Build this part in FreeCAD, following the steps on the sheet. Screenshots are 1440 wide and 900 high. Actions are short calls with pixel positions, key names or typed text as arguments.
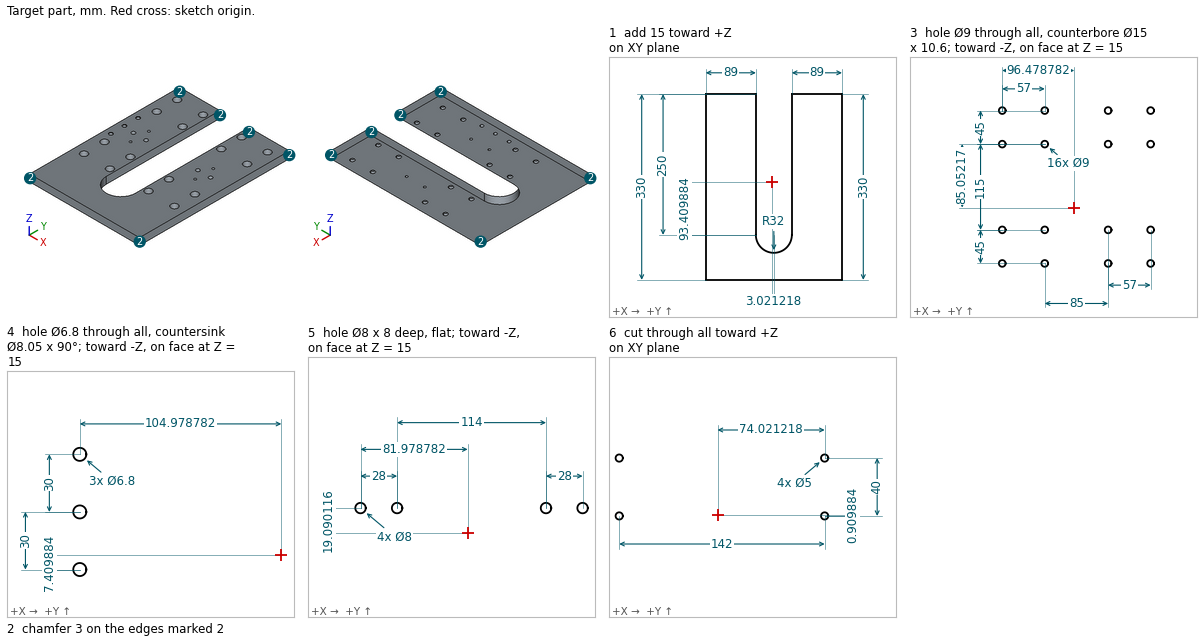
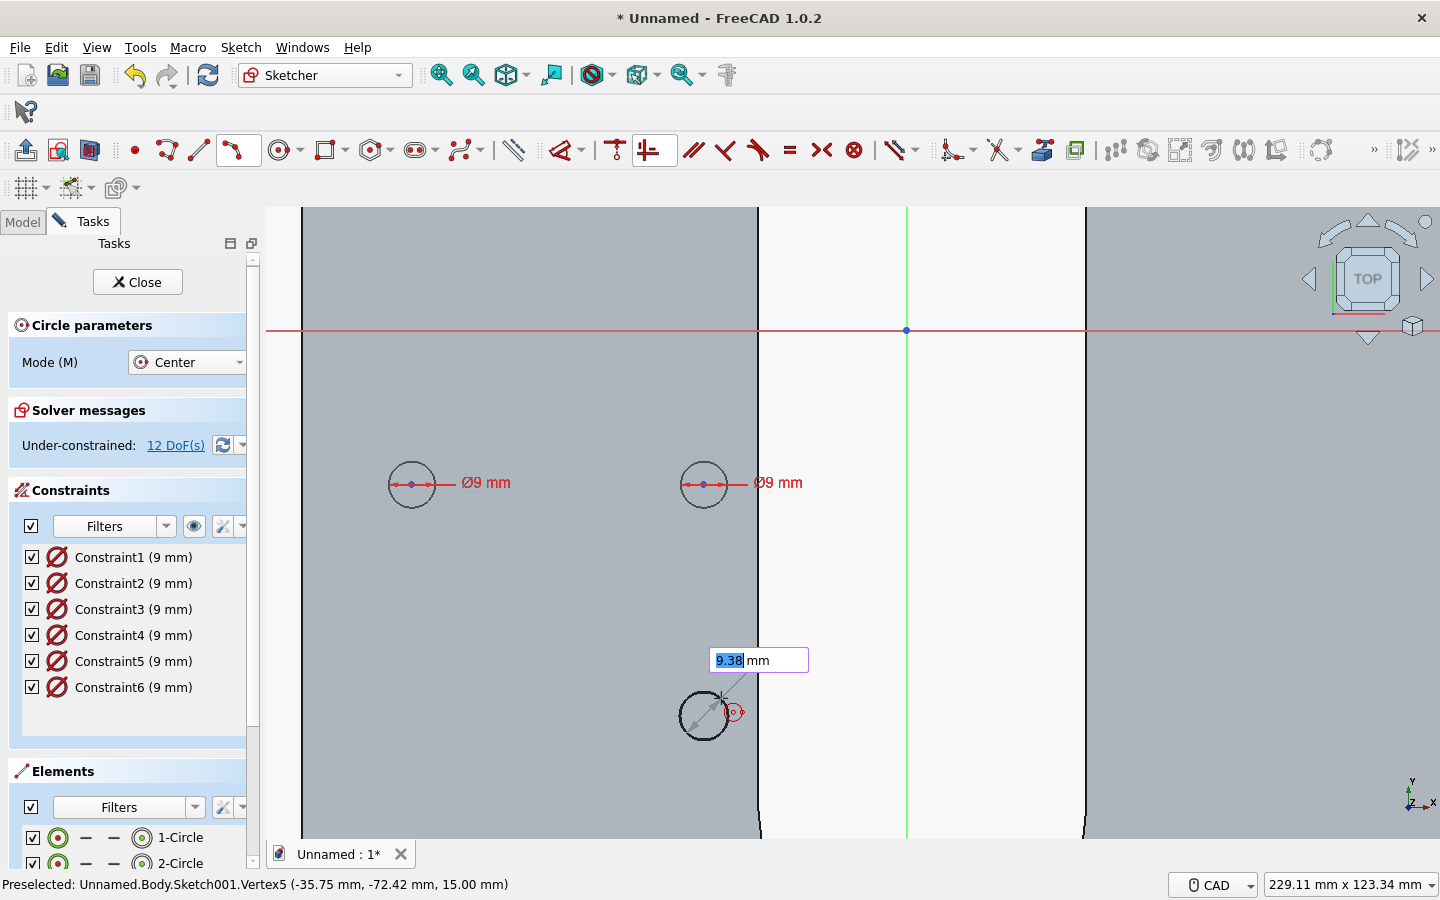
text(9)
key(Return)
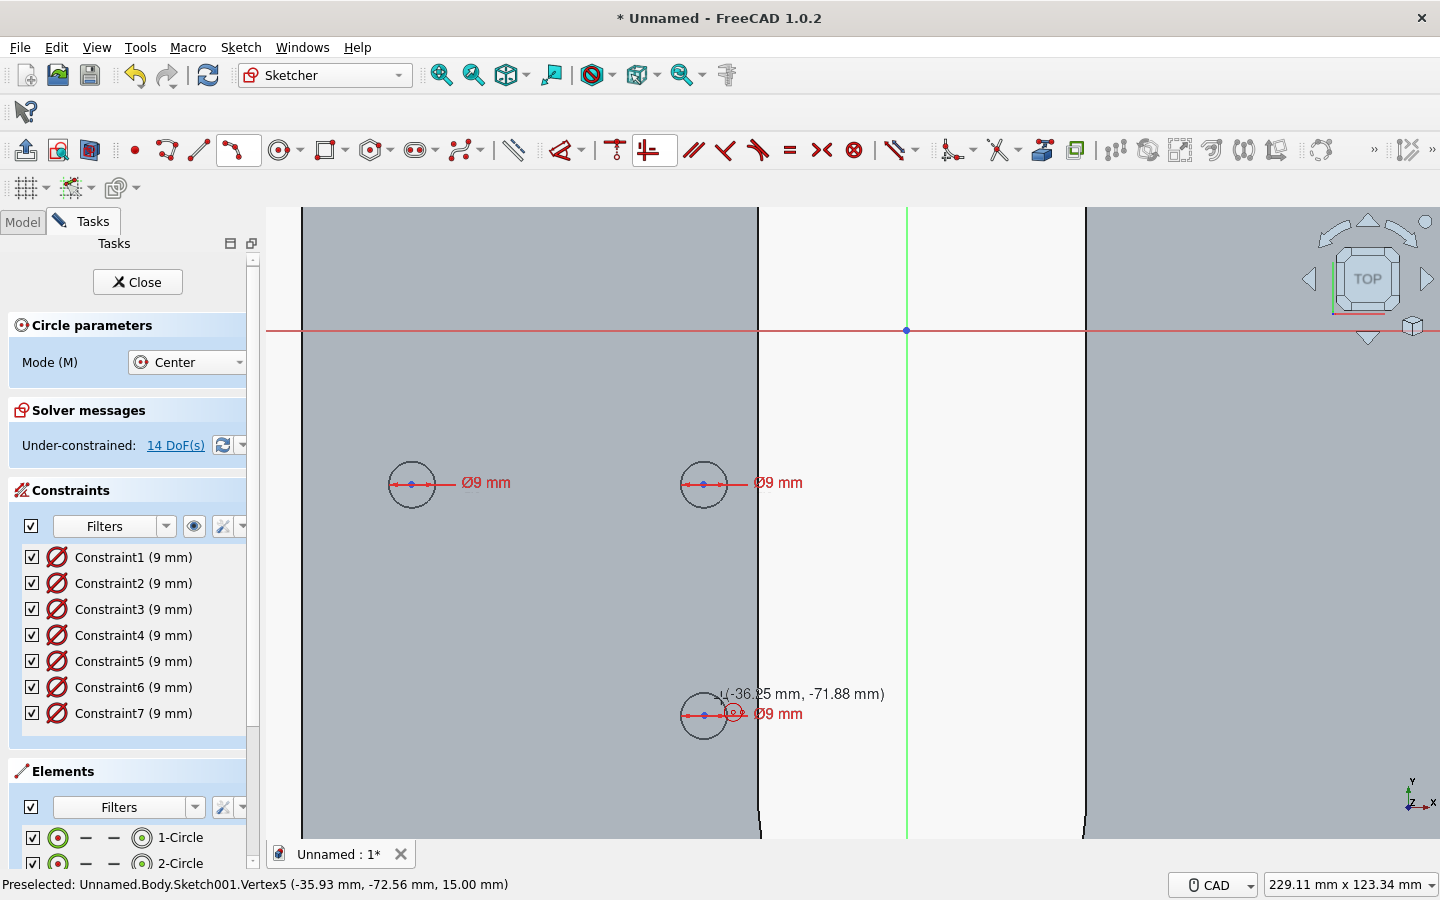
click(412, 715)
move(429, 698)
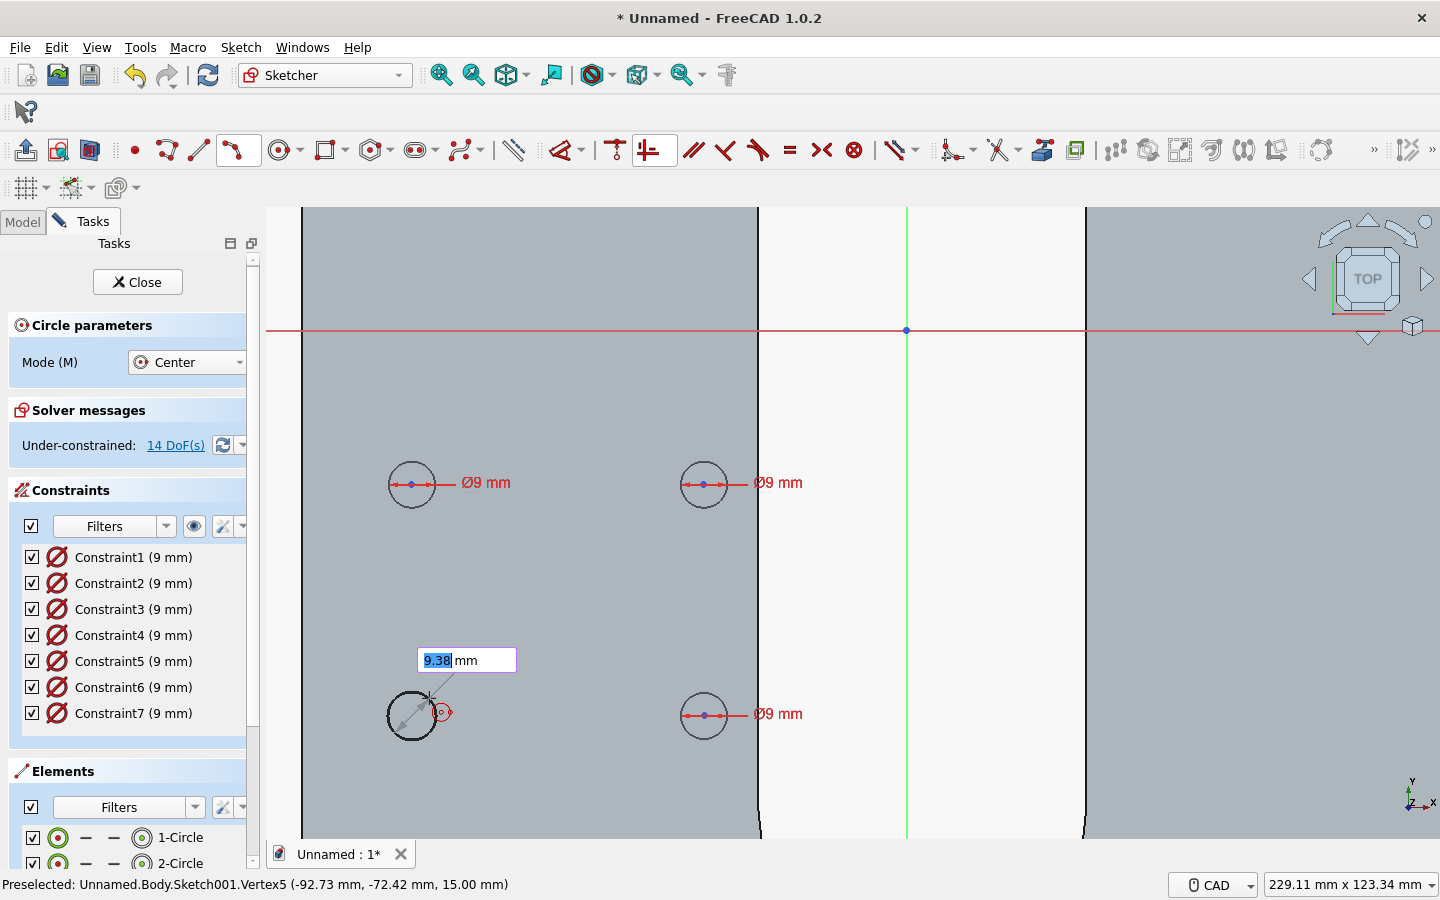
text(9)
key(Return)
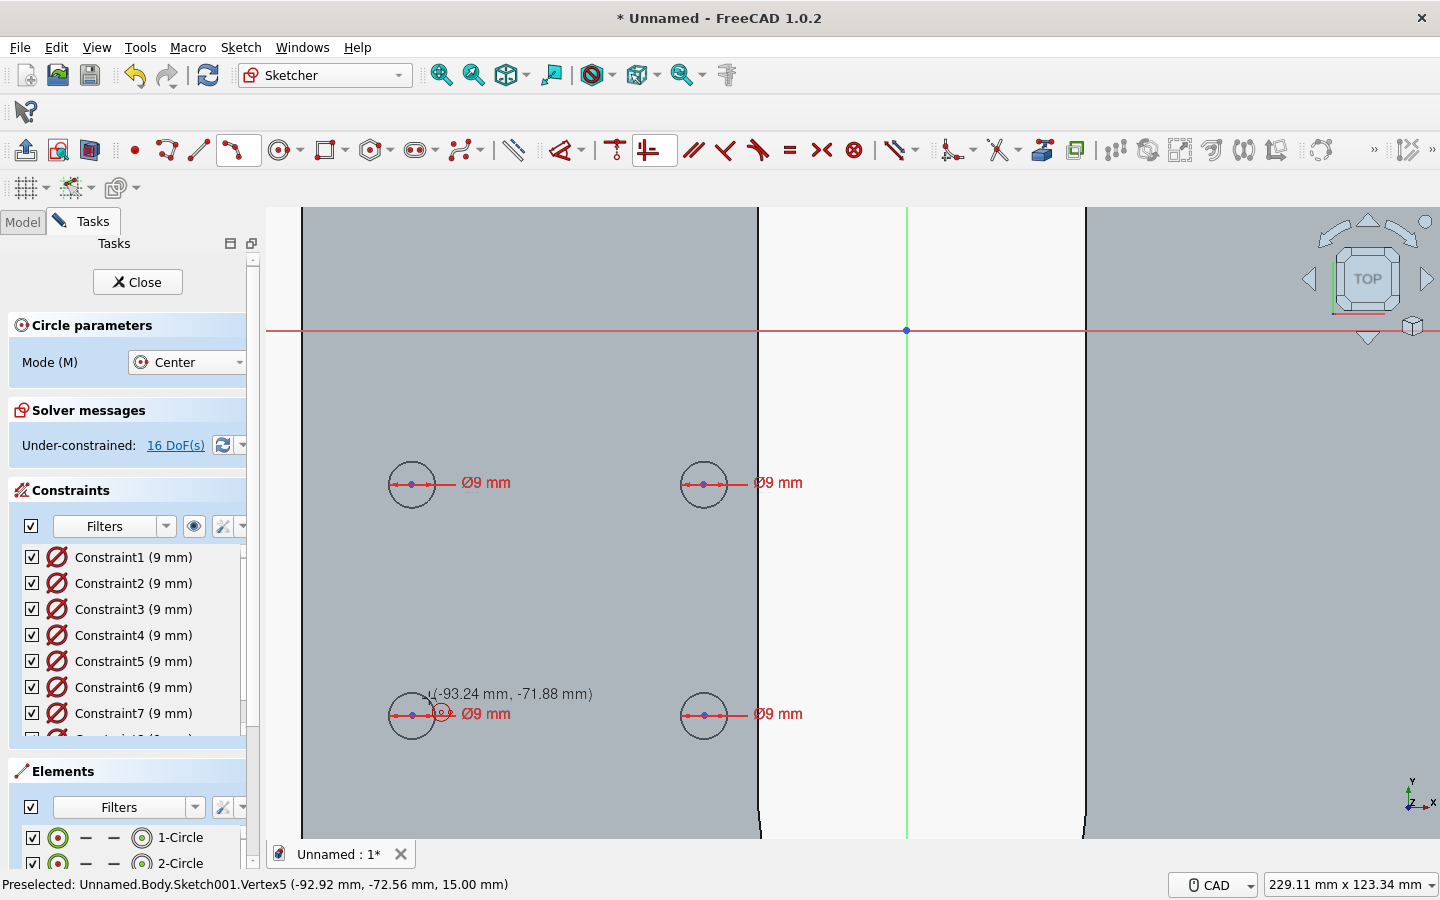
click(1140, 715)
move(1156, 698)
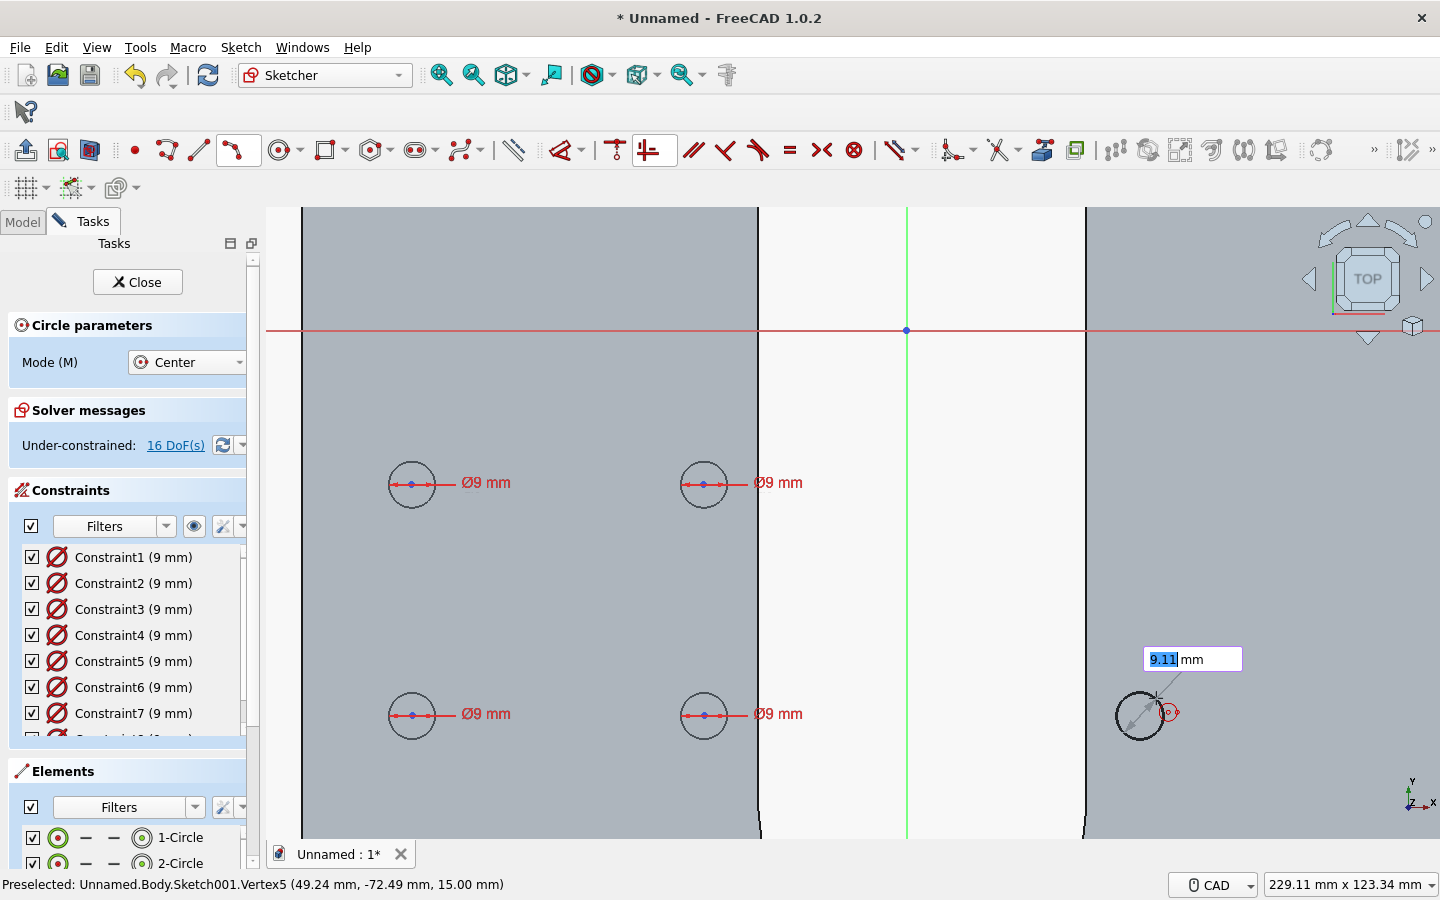
text(9)
key(Return)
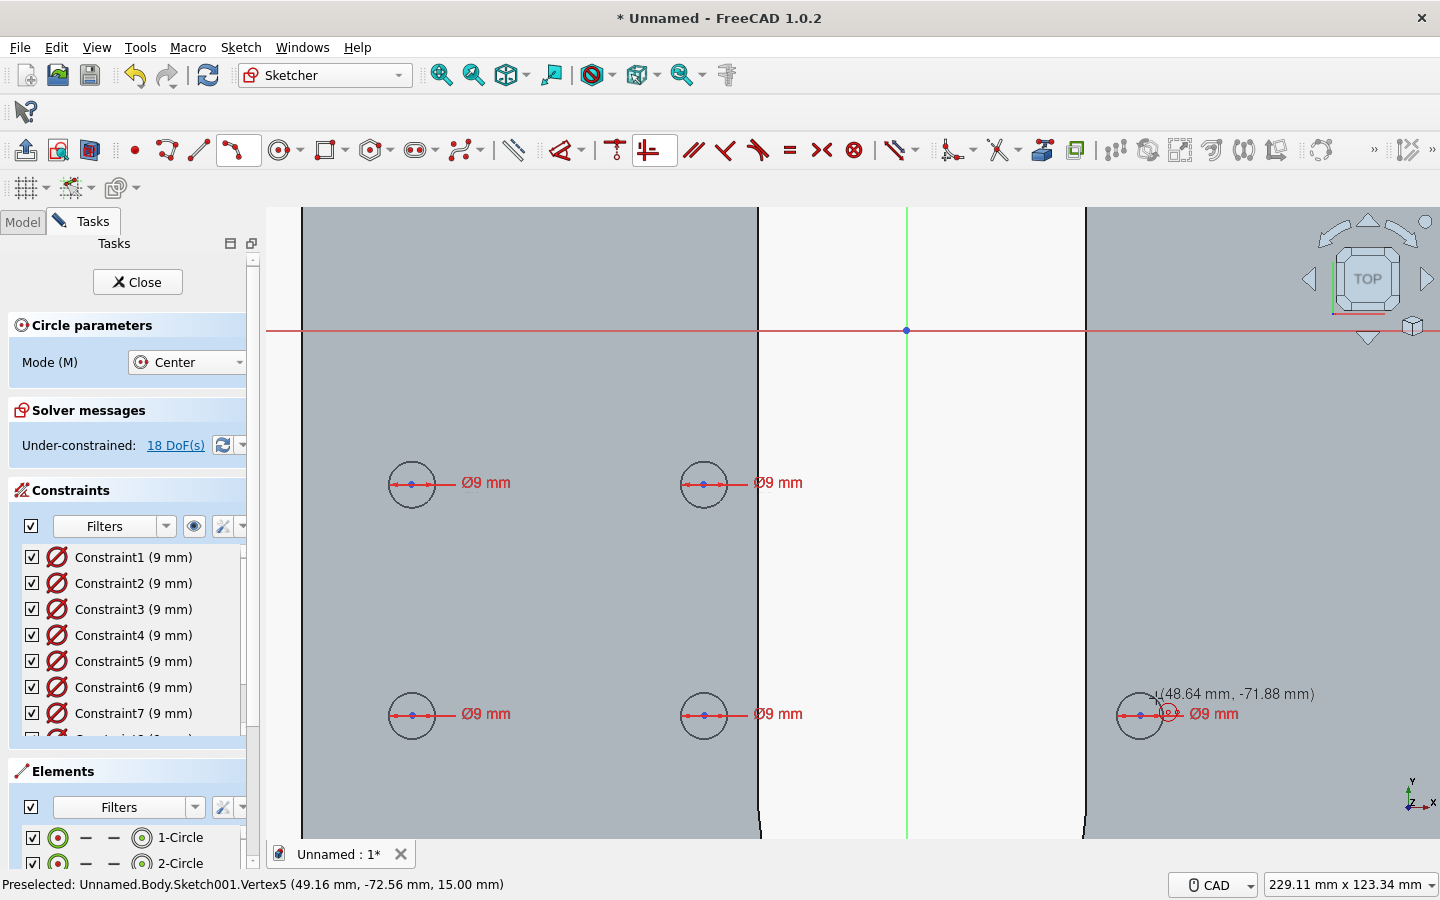
click(1140, 484)
move(1156, 468)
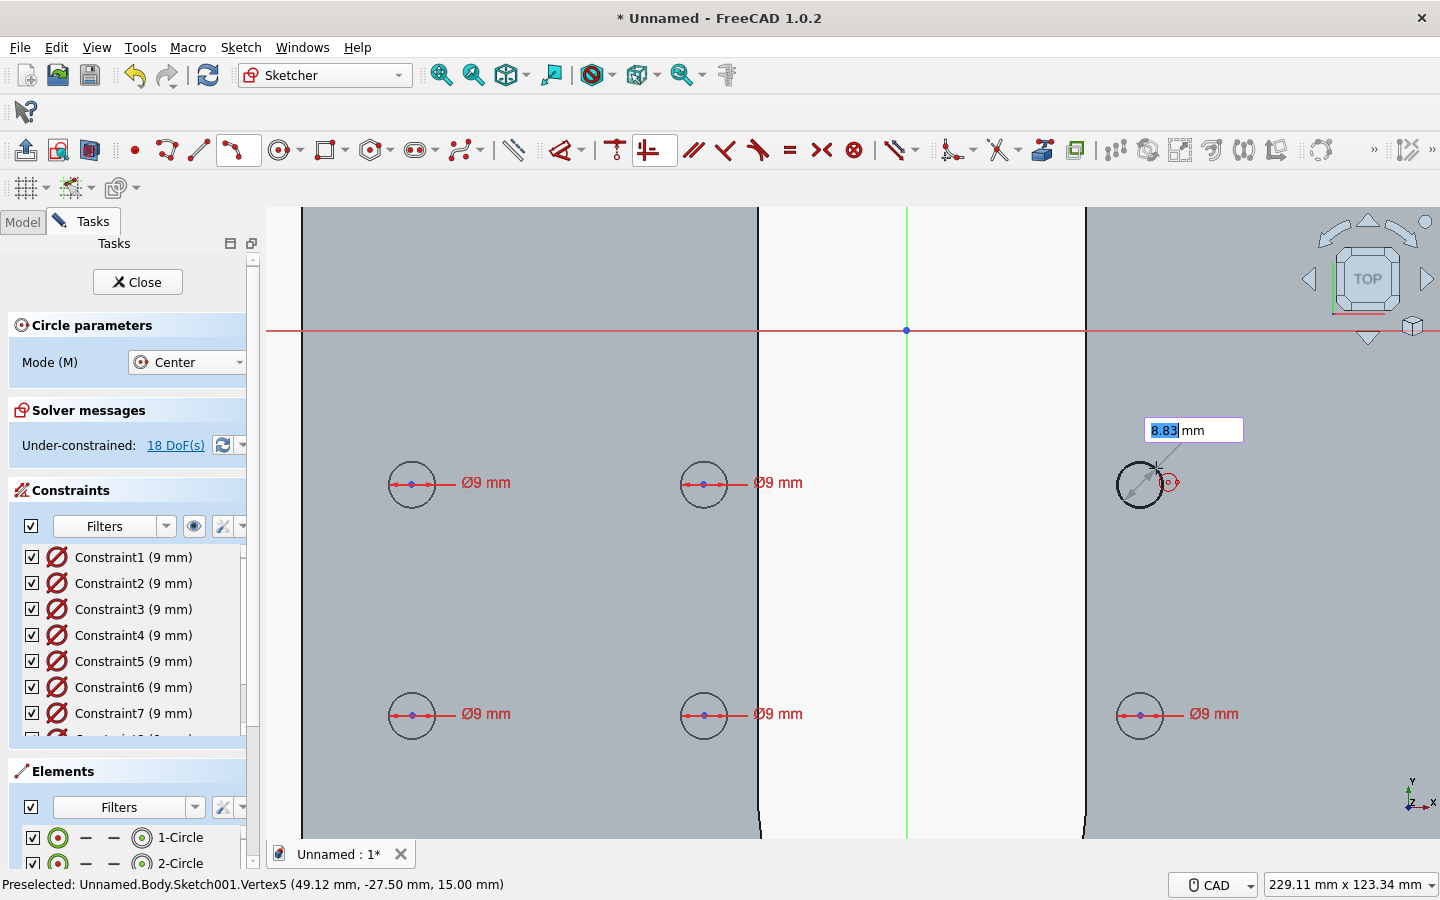
text(9)
key(Return)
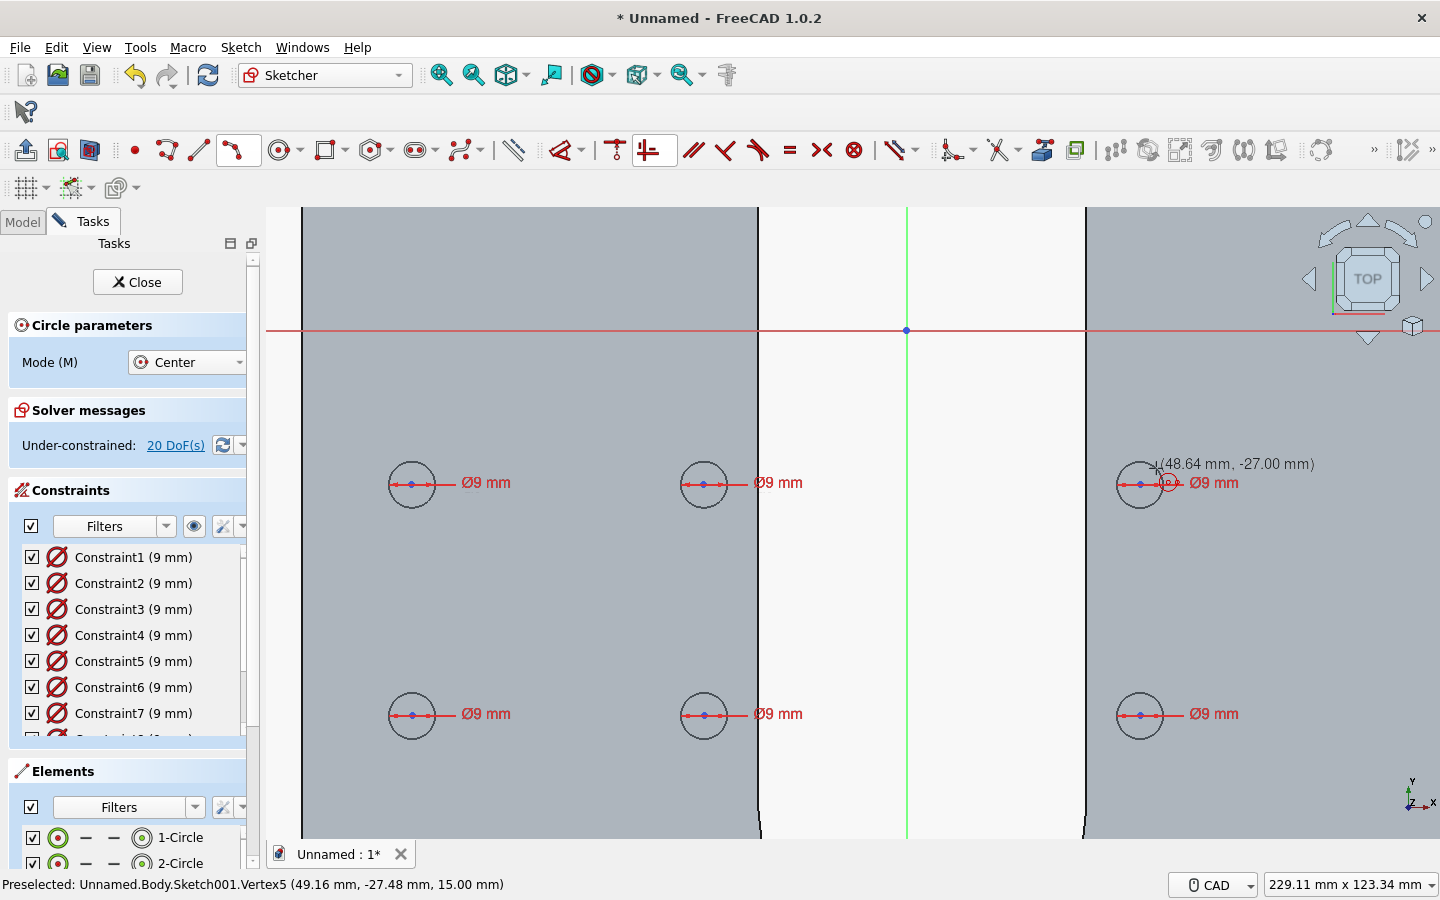
scroll(704, 717, down, 5)